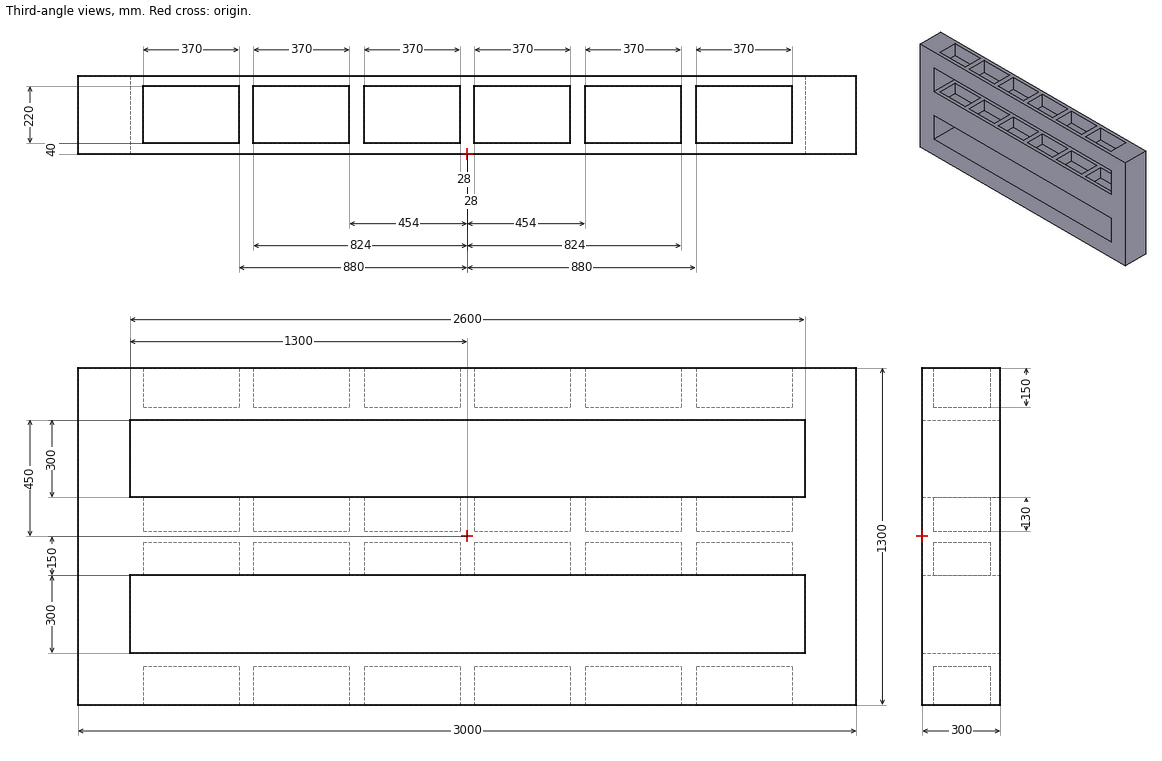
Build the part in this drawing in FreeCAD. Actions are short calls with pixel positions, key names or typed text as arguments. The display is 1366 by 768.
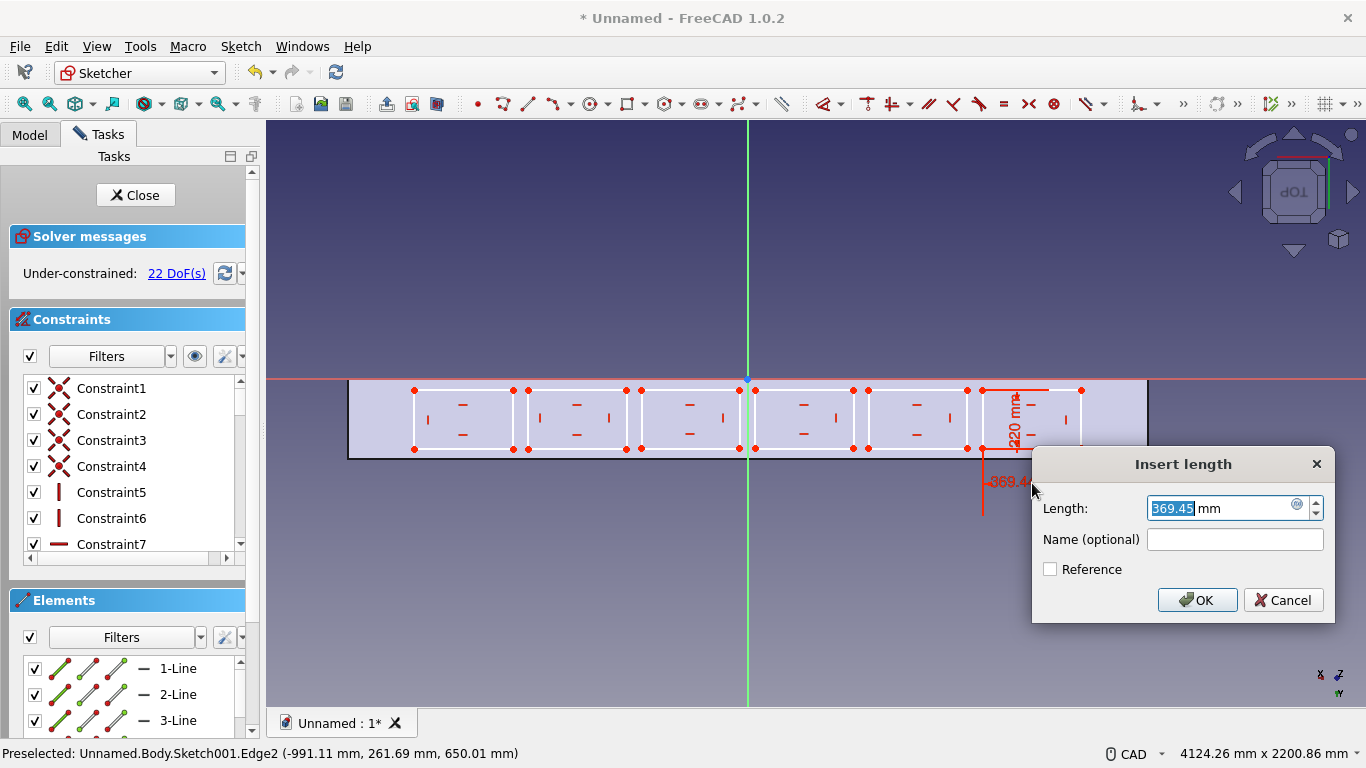
text(370)
key(Return)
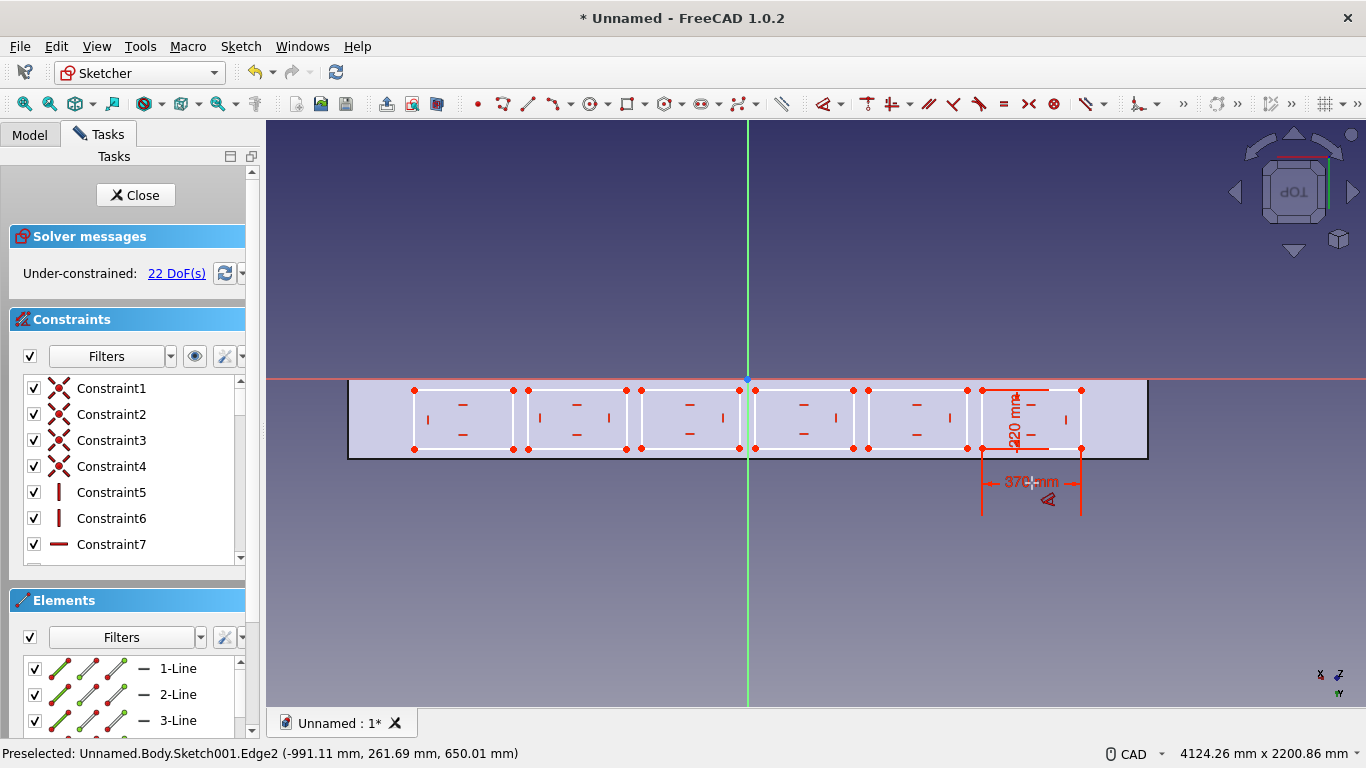
click(414, 408)
click(380, 420)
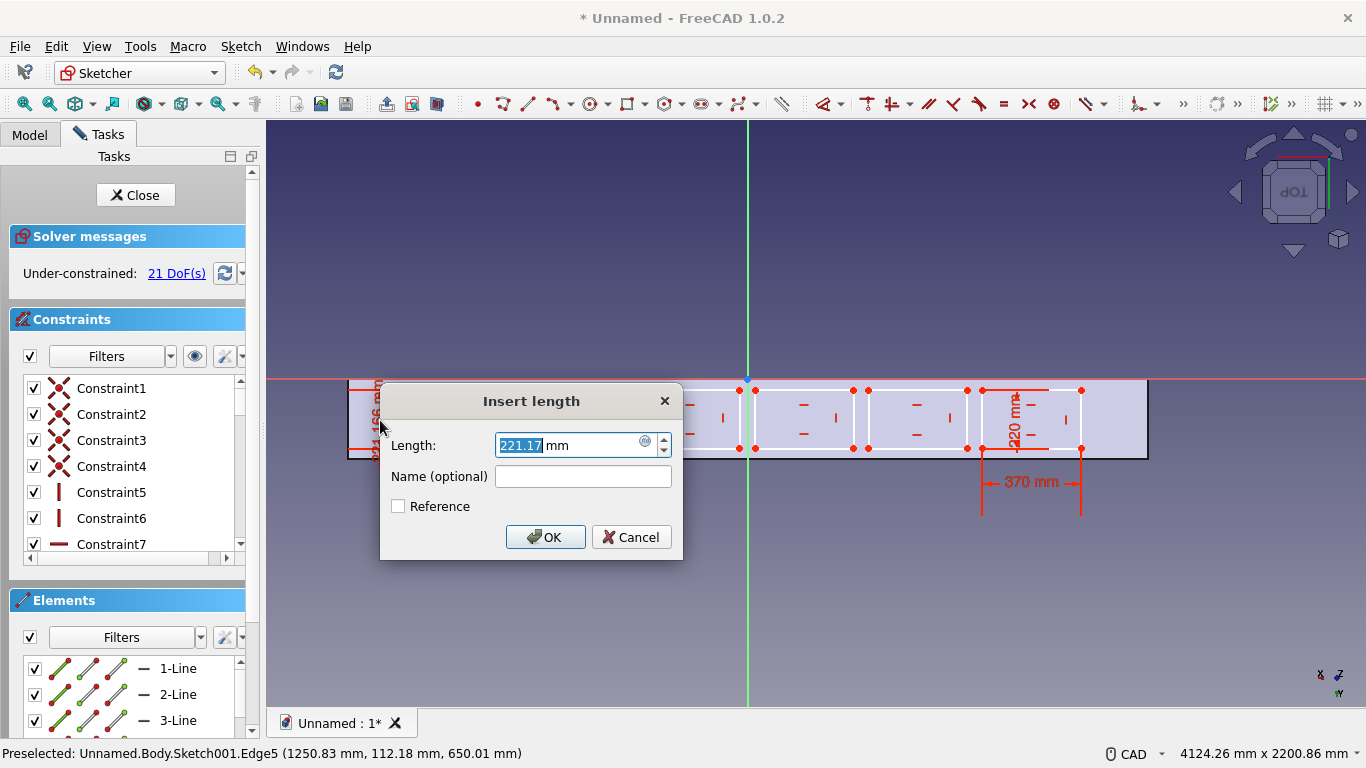
text(220)
key(Return)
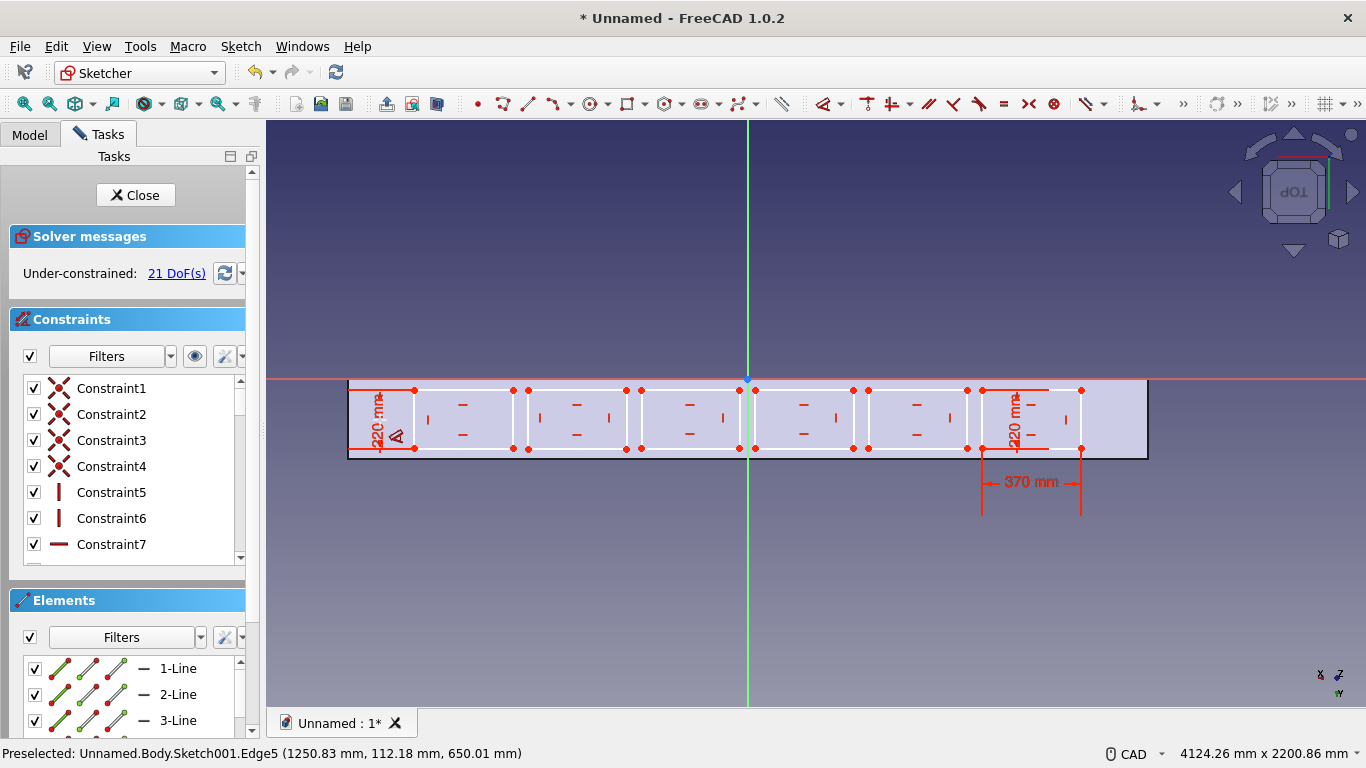
click(444, 449)
click(464, 483)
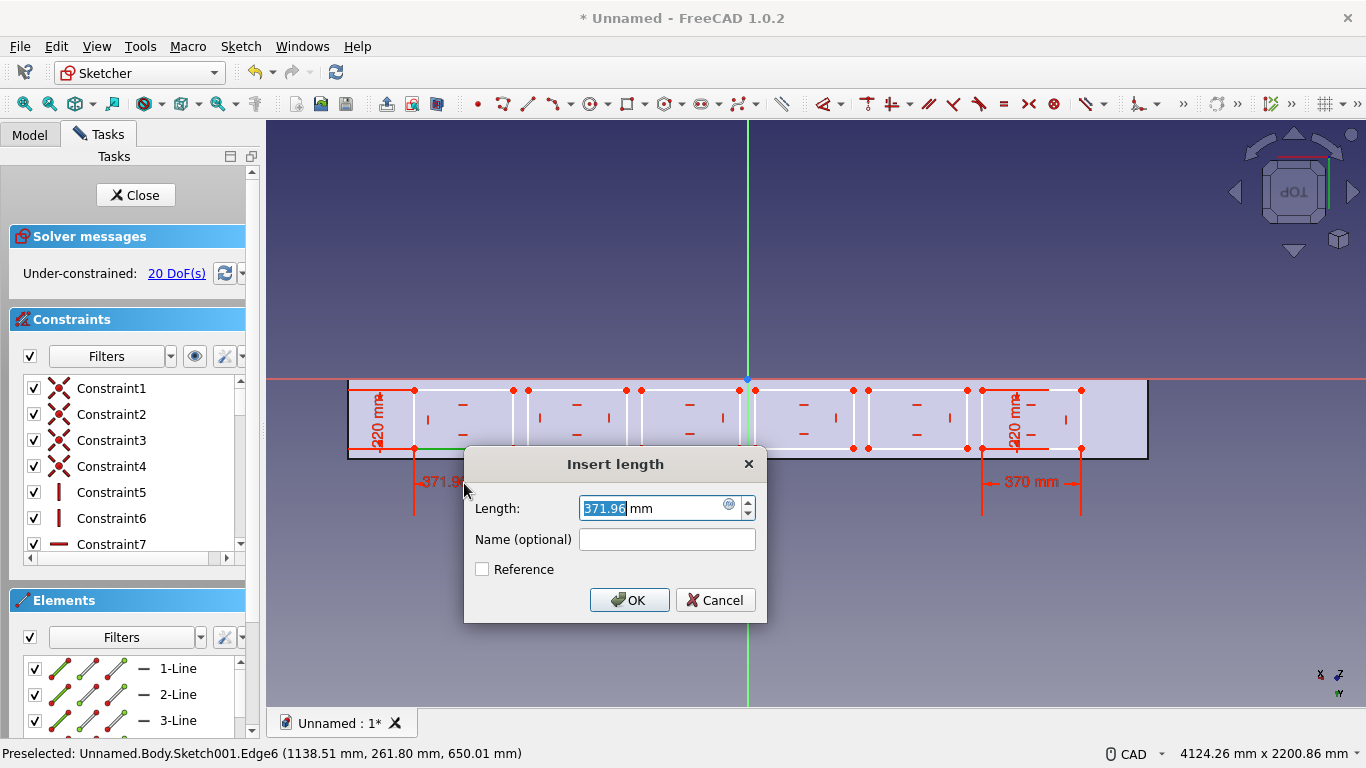
text(370)
key(Return)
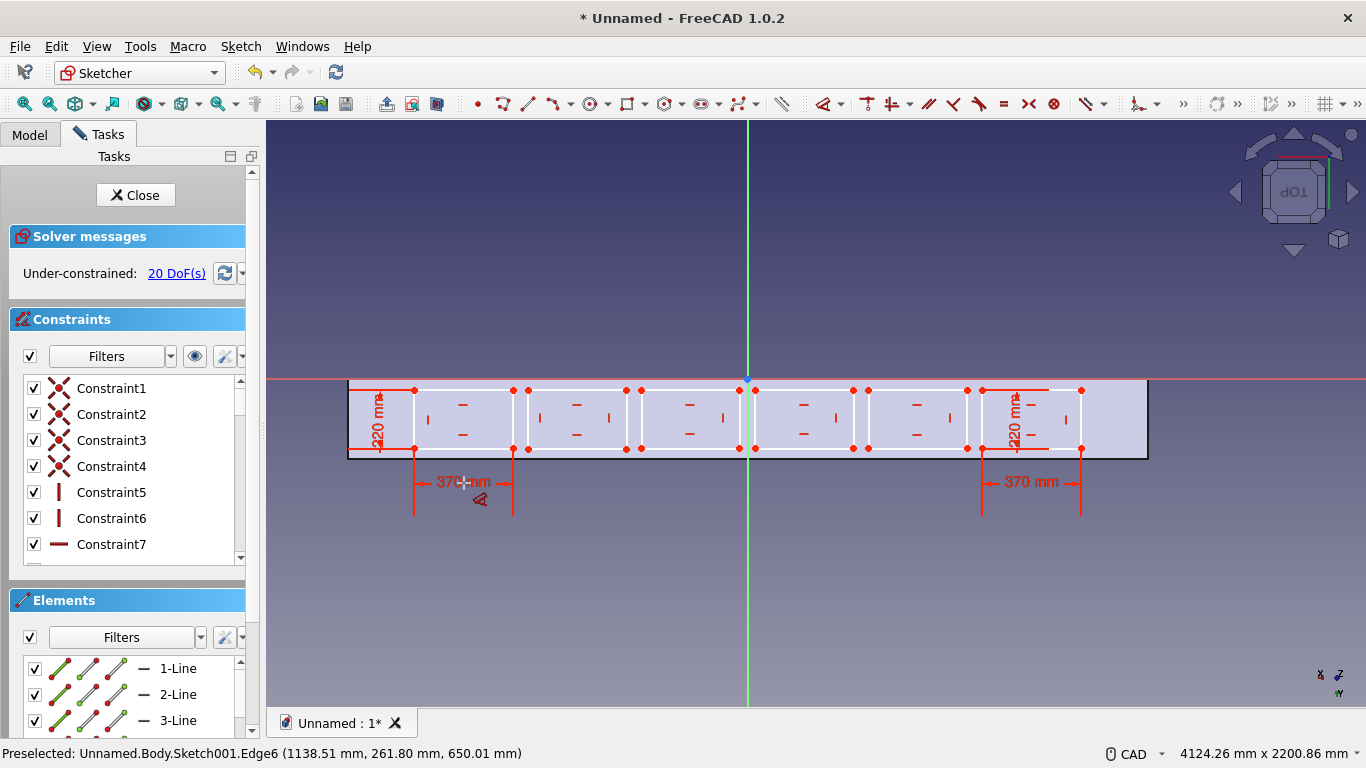
click(869, 408)
click(903, 420)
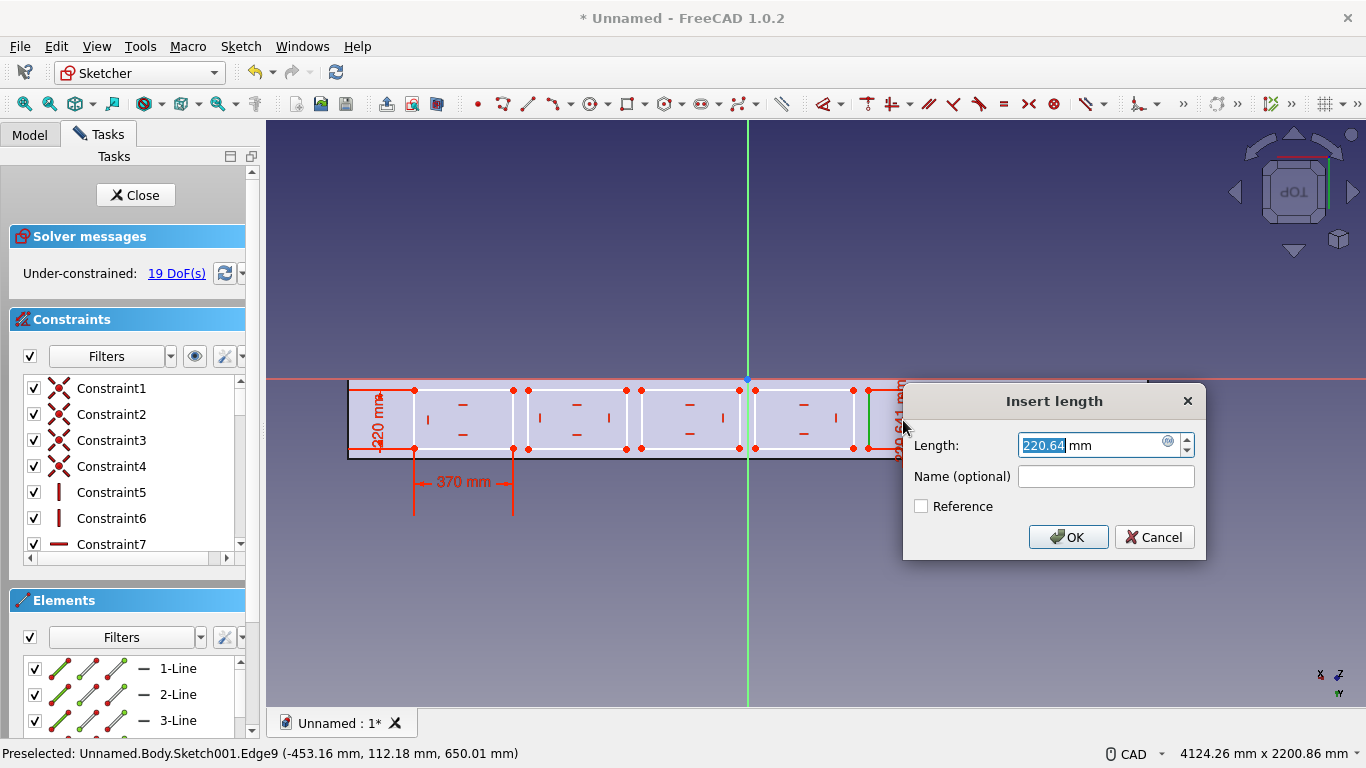
text(220)
key(Return)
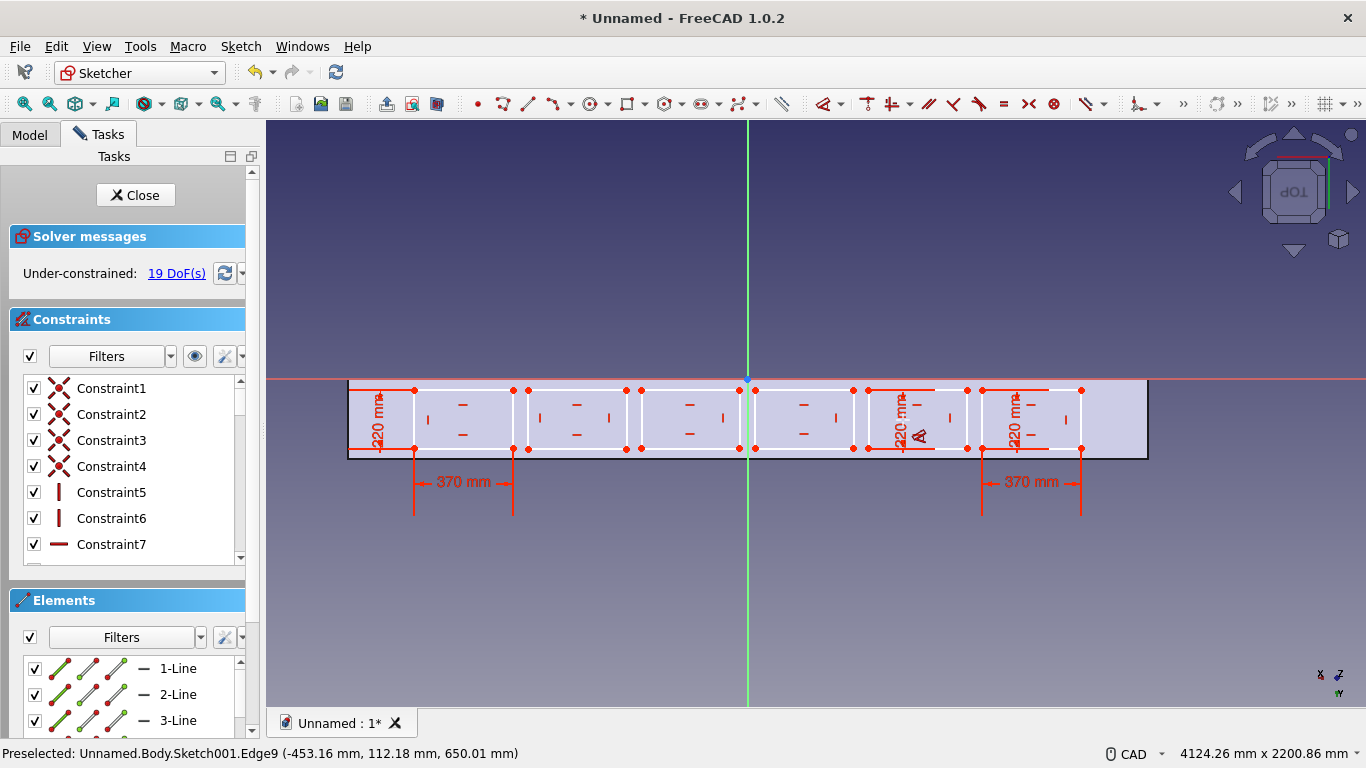
click(898, 449)
click(918, 483)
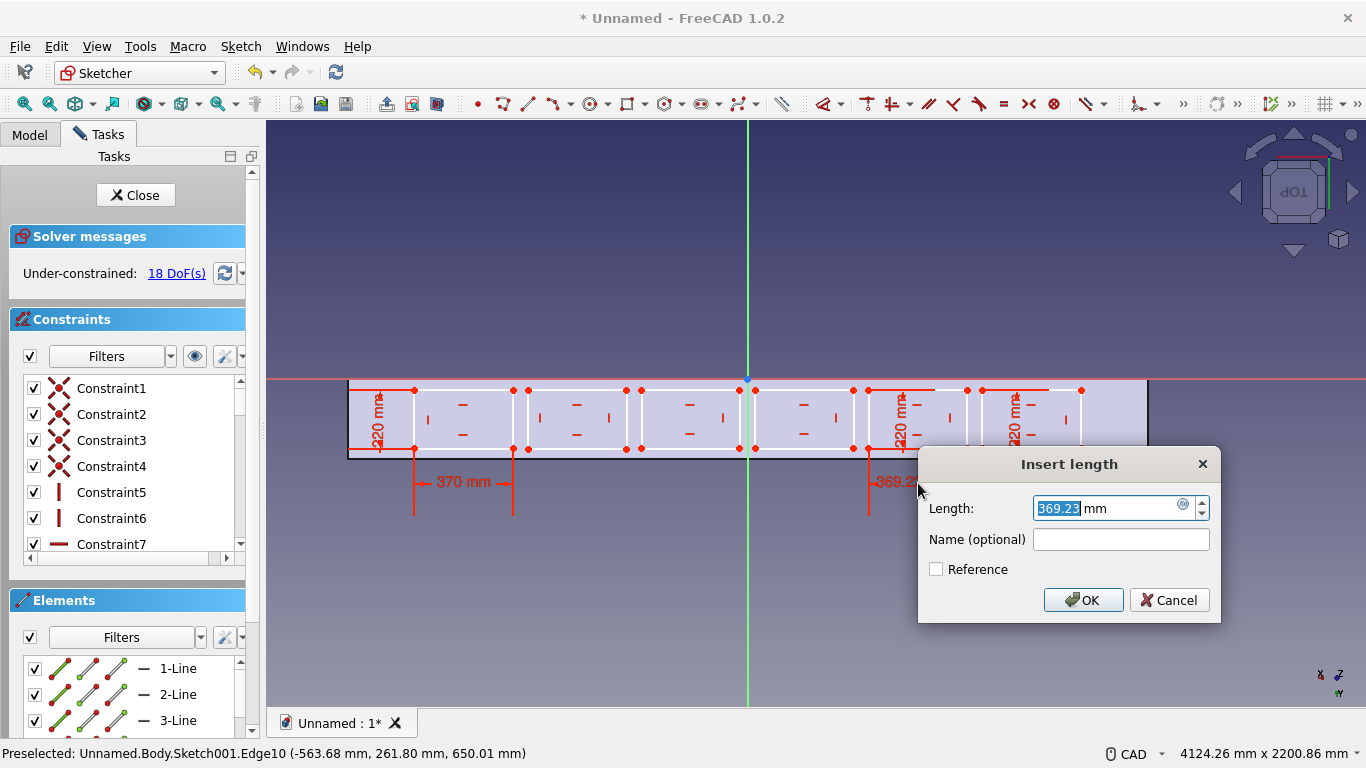
text(370)
key(Return)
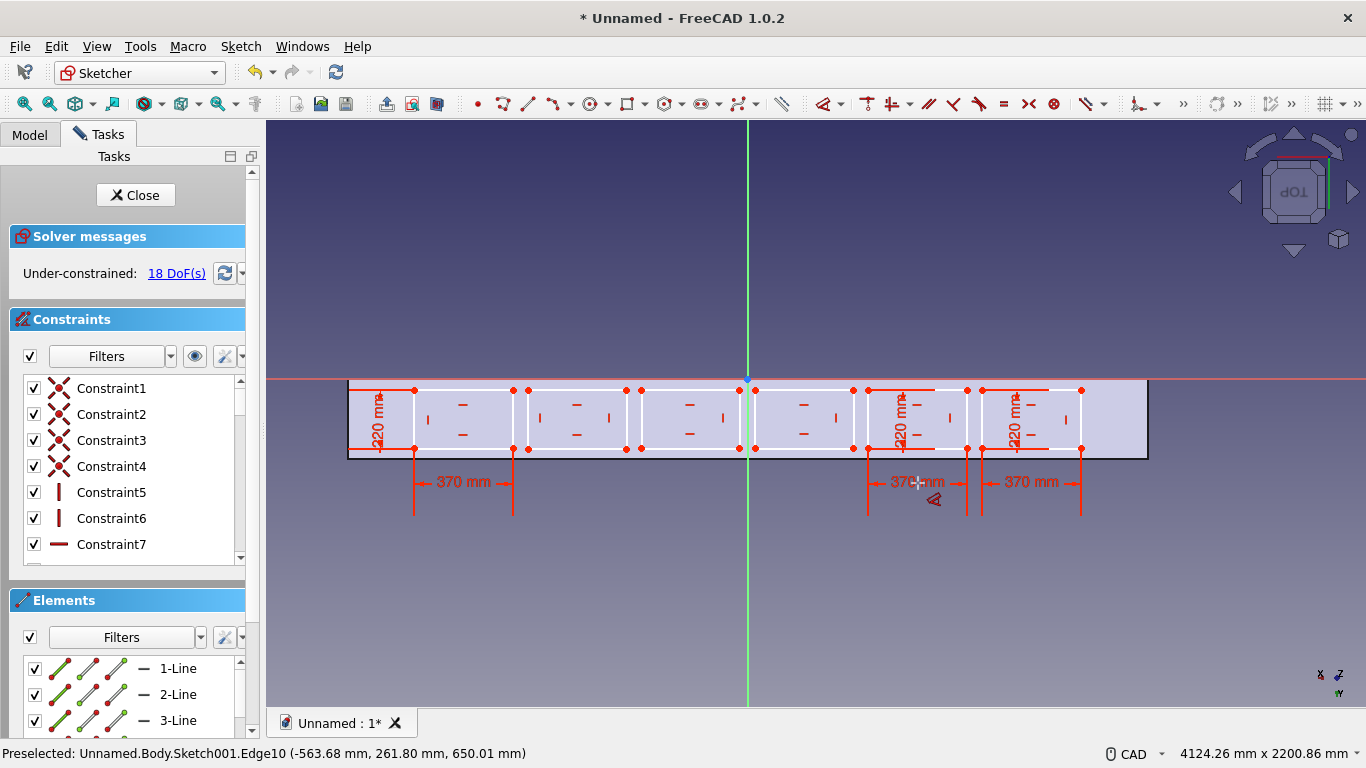
scroll(755, 408, up, 3)